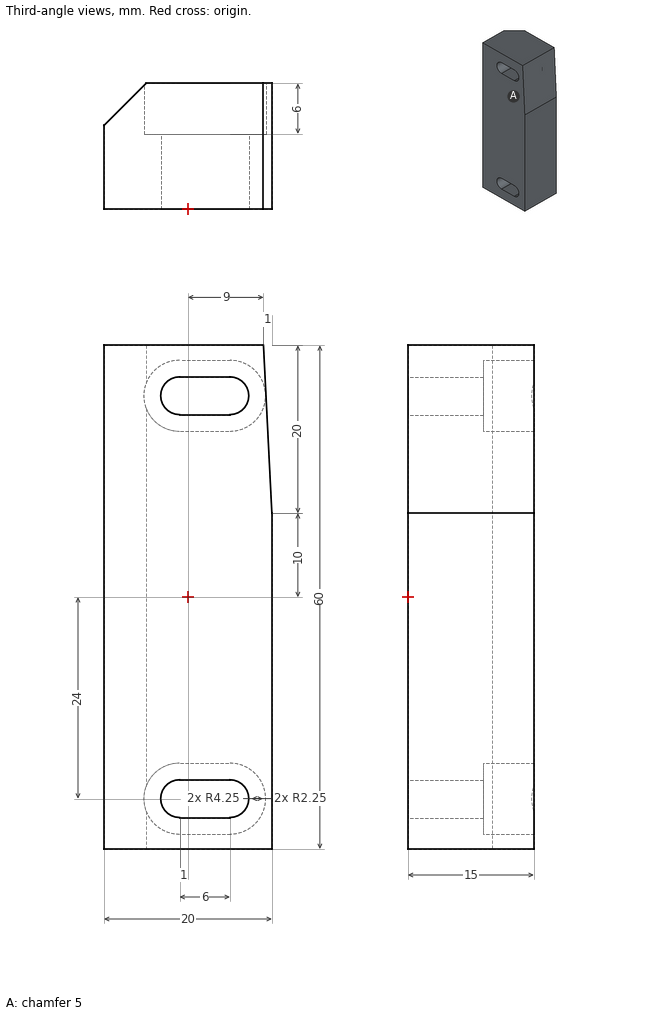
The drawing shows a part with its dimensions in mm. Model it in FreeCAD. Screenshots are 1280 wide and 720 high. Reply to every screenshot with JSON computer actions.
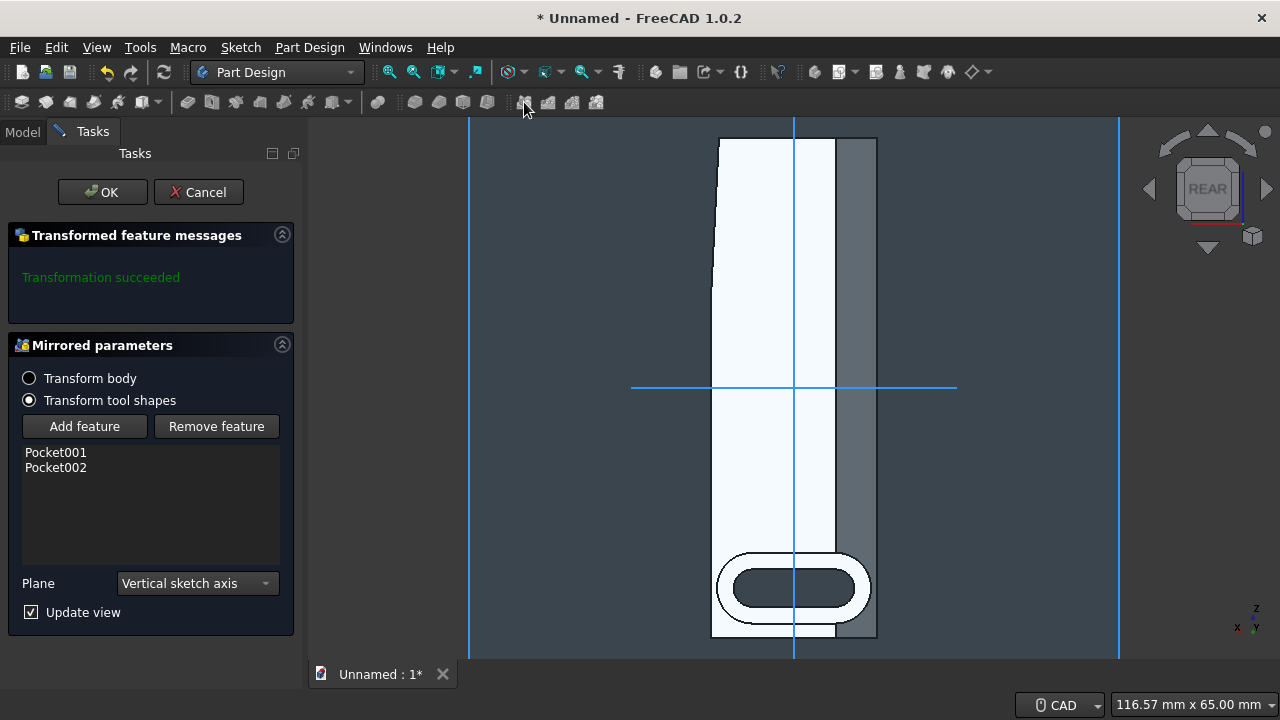
{"action": "left_click", "coordinate": [198, 584]}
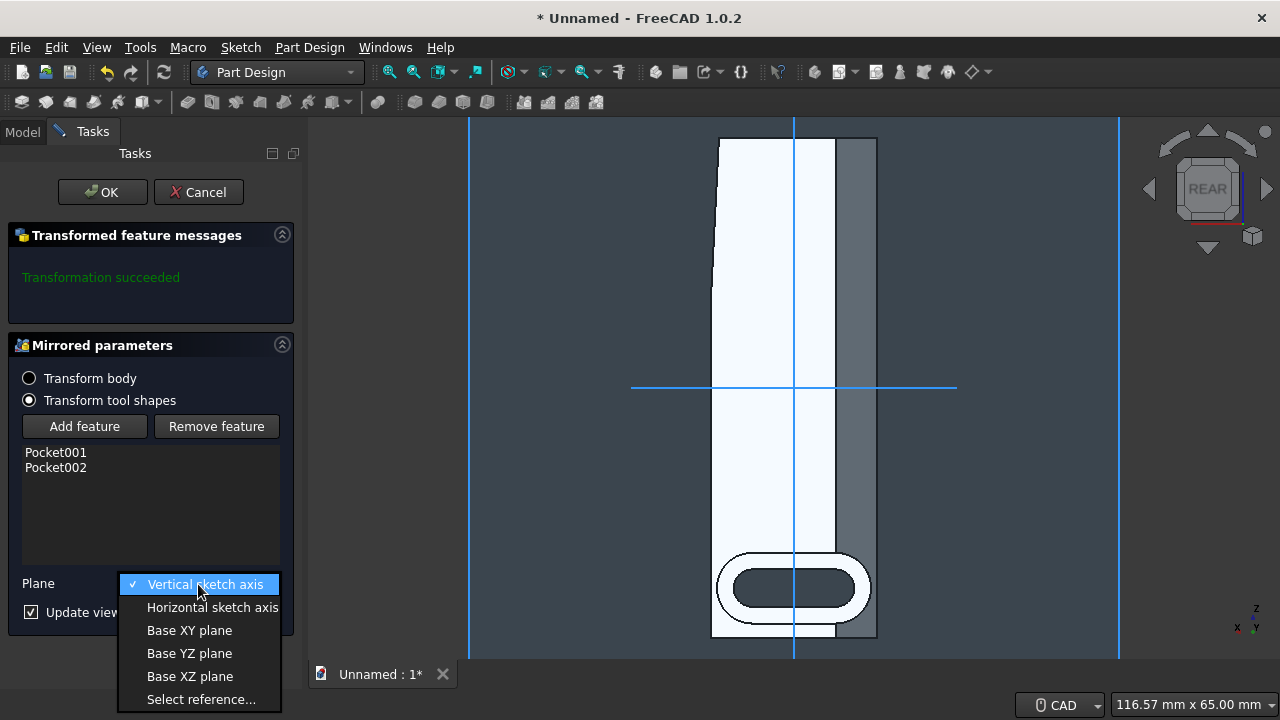
{"action": "left_click", "coordinate": [198, 630]}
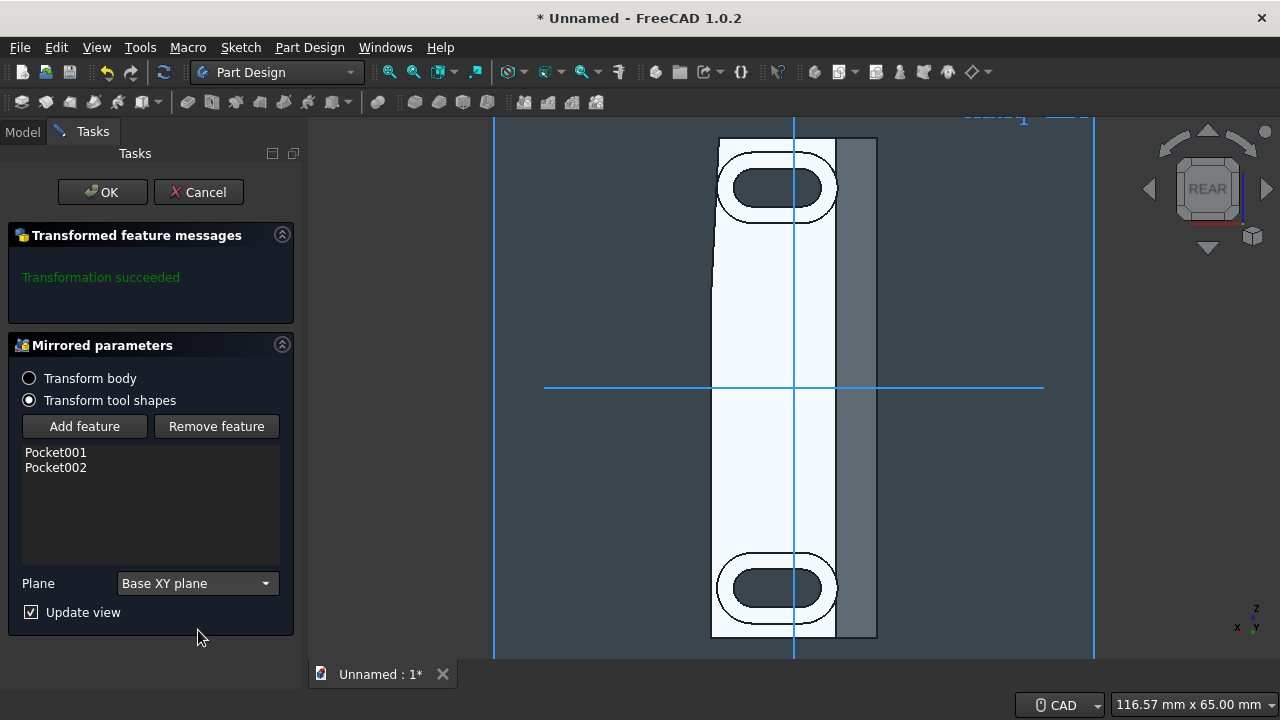
{"action": "left_click", "coordinate": [103, 192]}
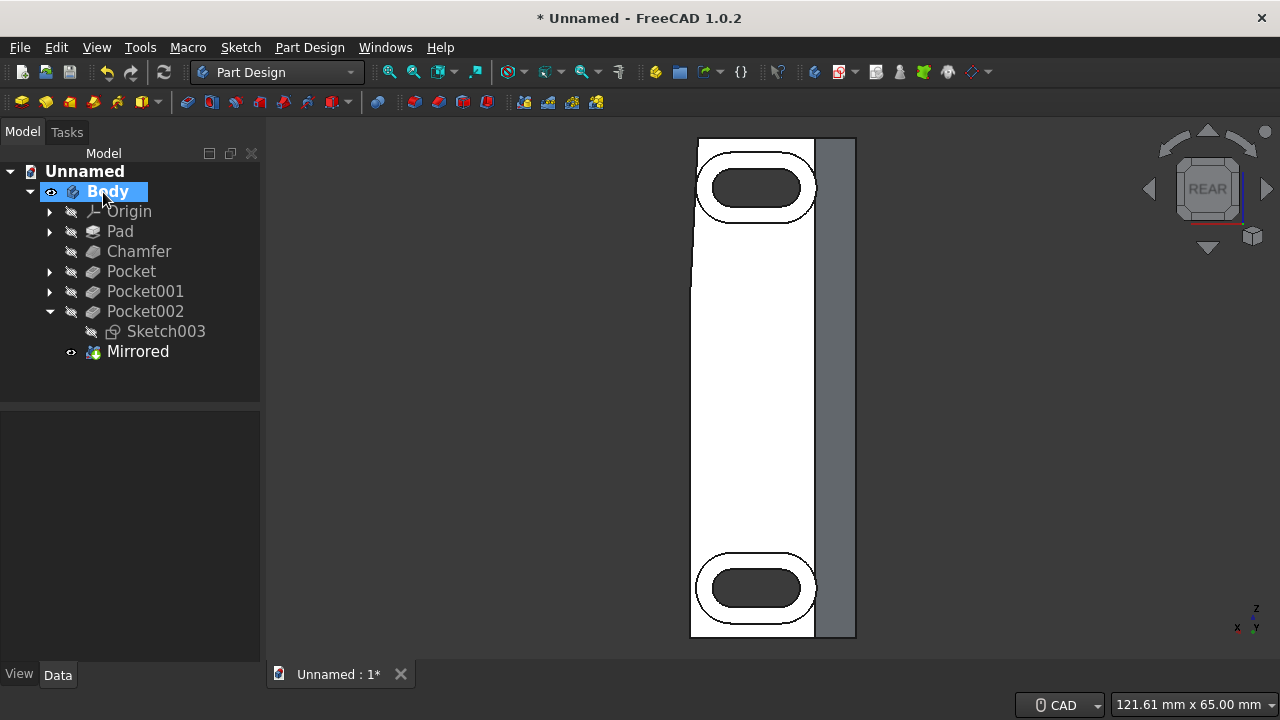
{"action": "key", "text": "0"}